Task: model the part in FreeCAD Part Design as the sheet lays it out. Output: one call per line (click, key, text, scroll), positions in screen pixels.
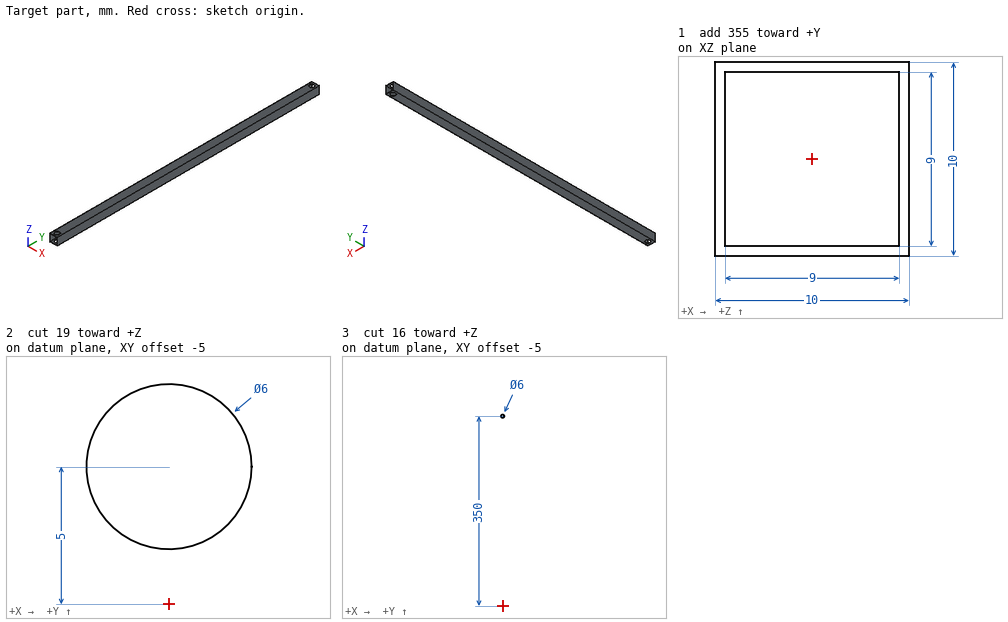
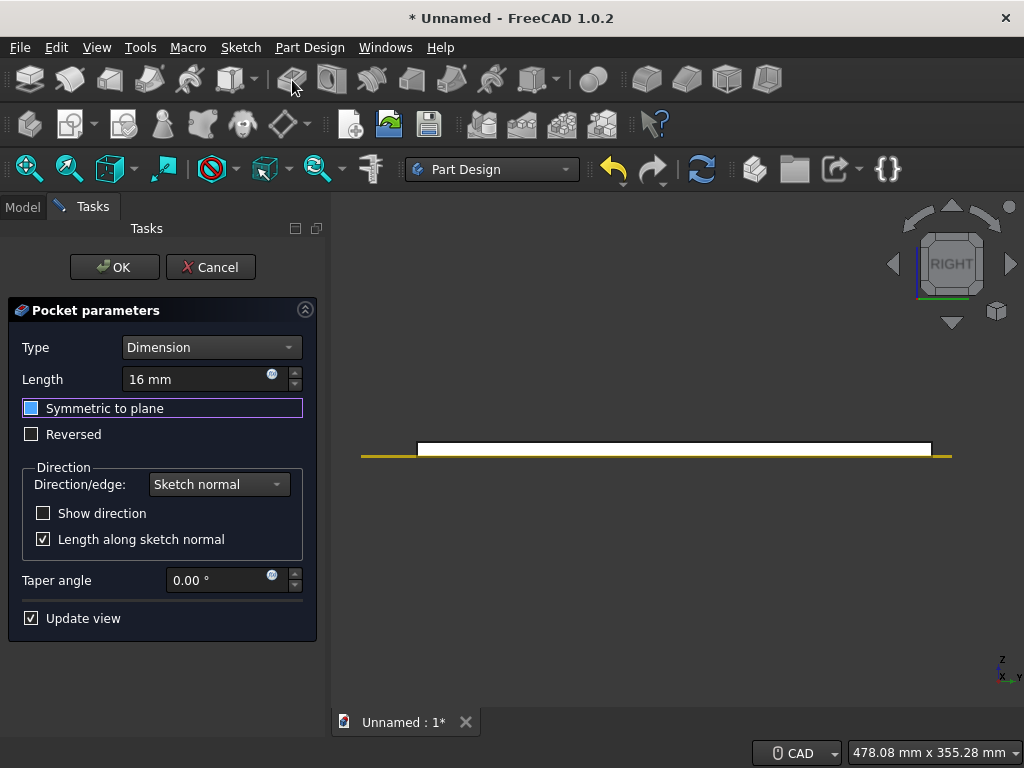
click(30, 434)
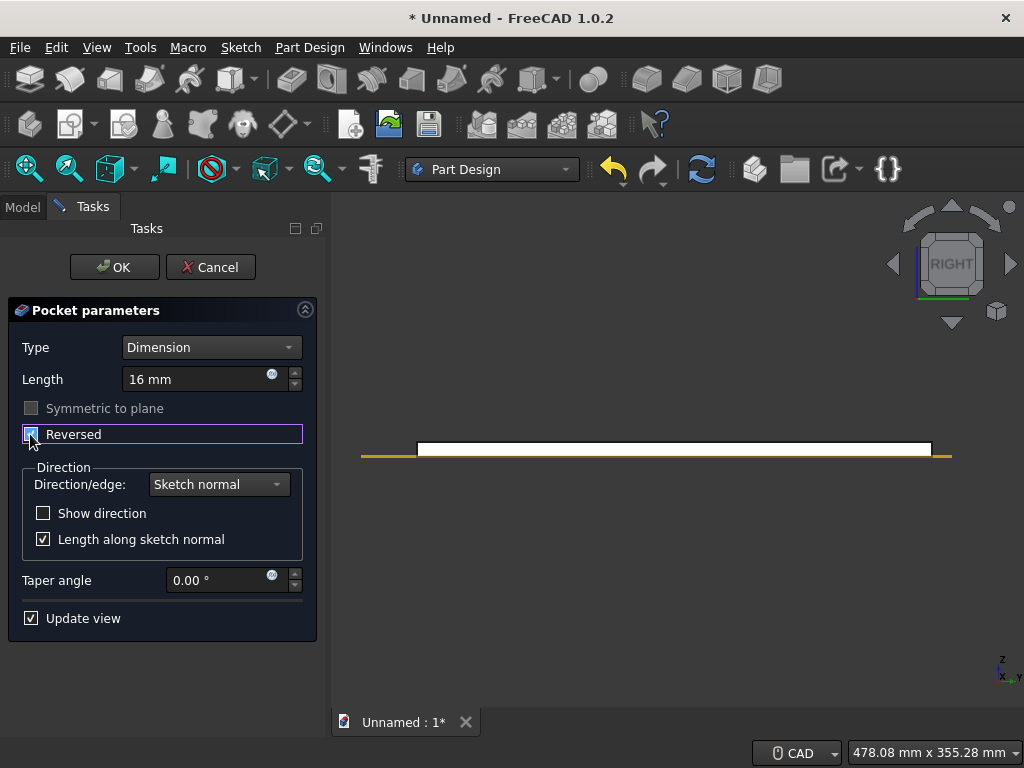
click(115, 267)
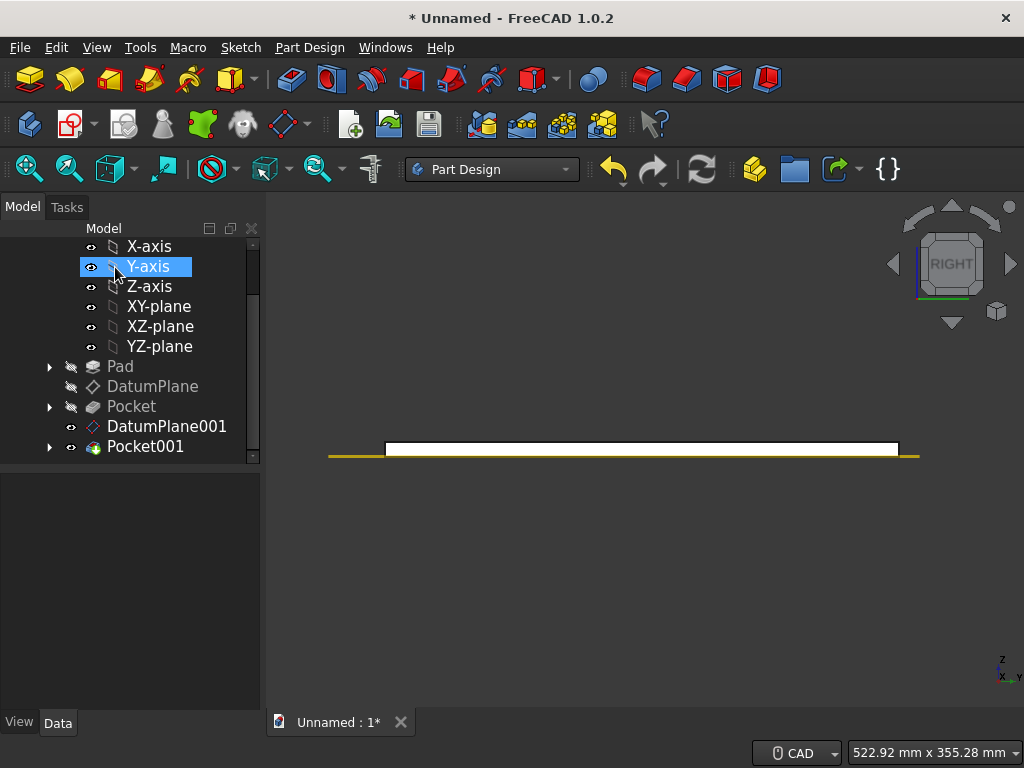
click(116, 427)
key(space)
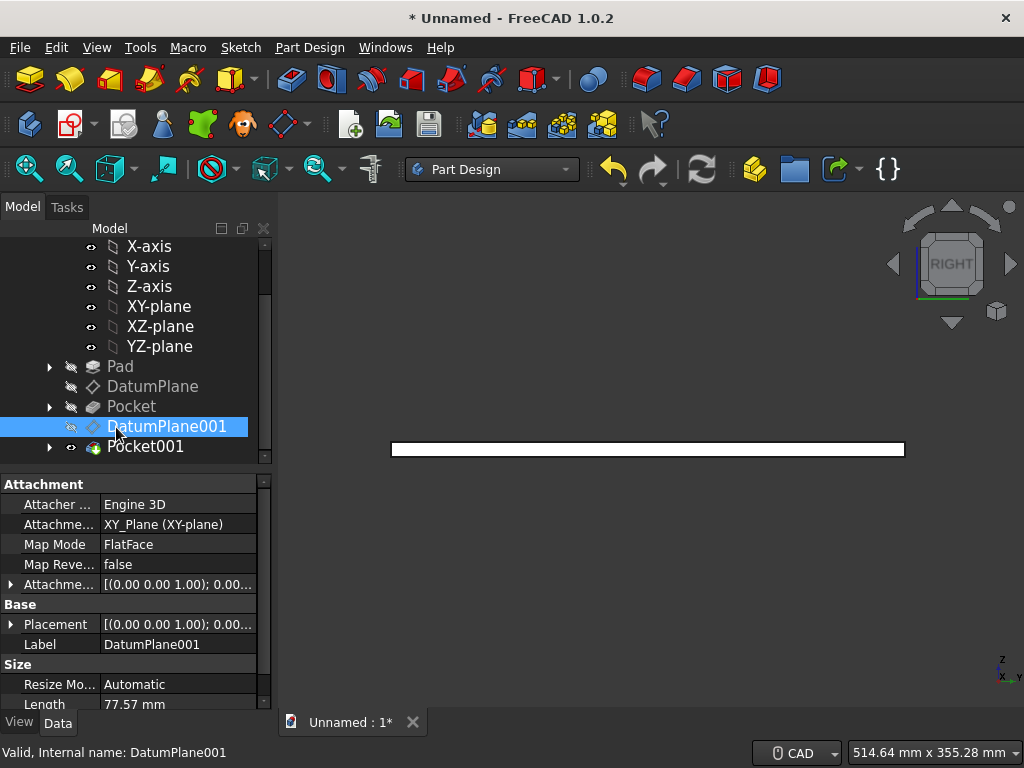
key(0)